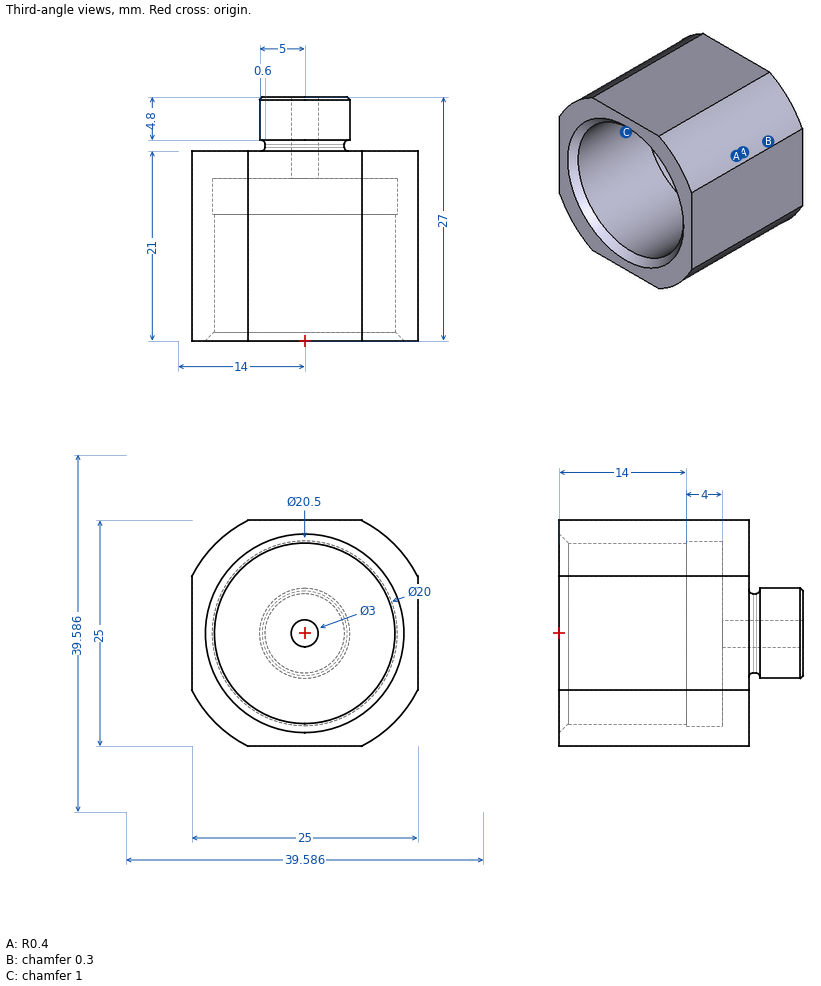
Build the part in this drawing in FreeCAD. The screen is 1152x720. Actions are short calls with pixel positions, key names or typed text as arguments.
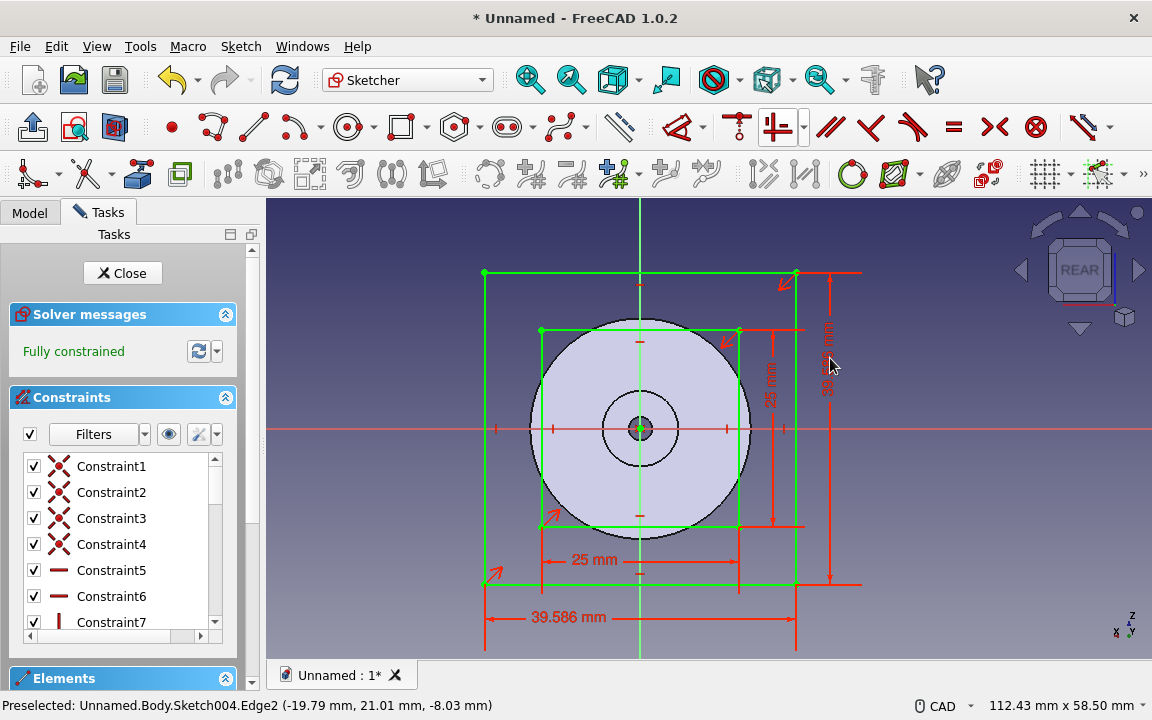
click(123, 273)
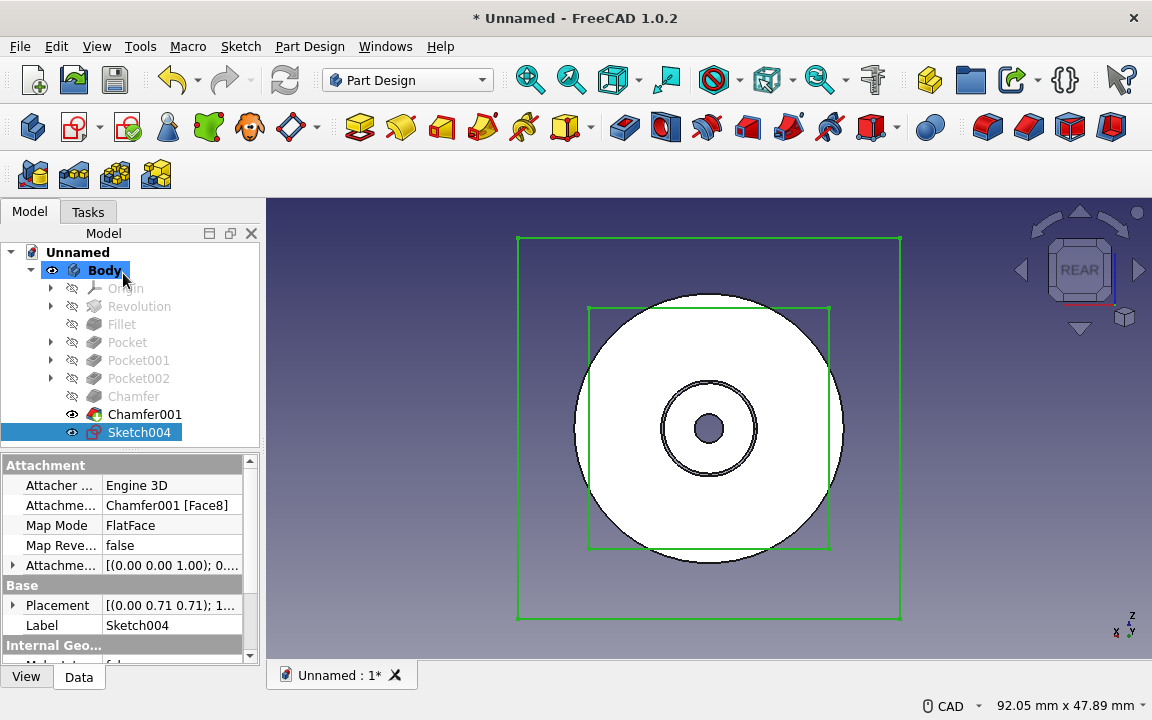
click(625, 128)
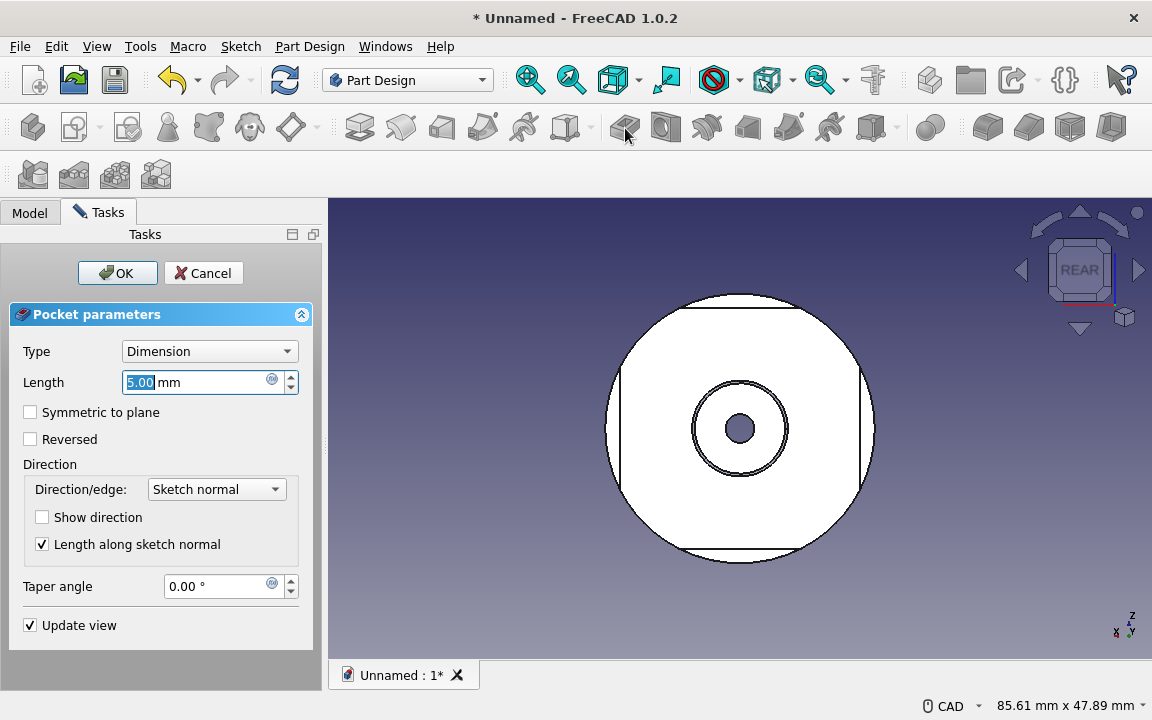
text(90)
key(Tab)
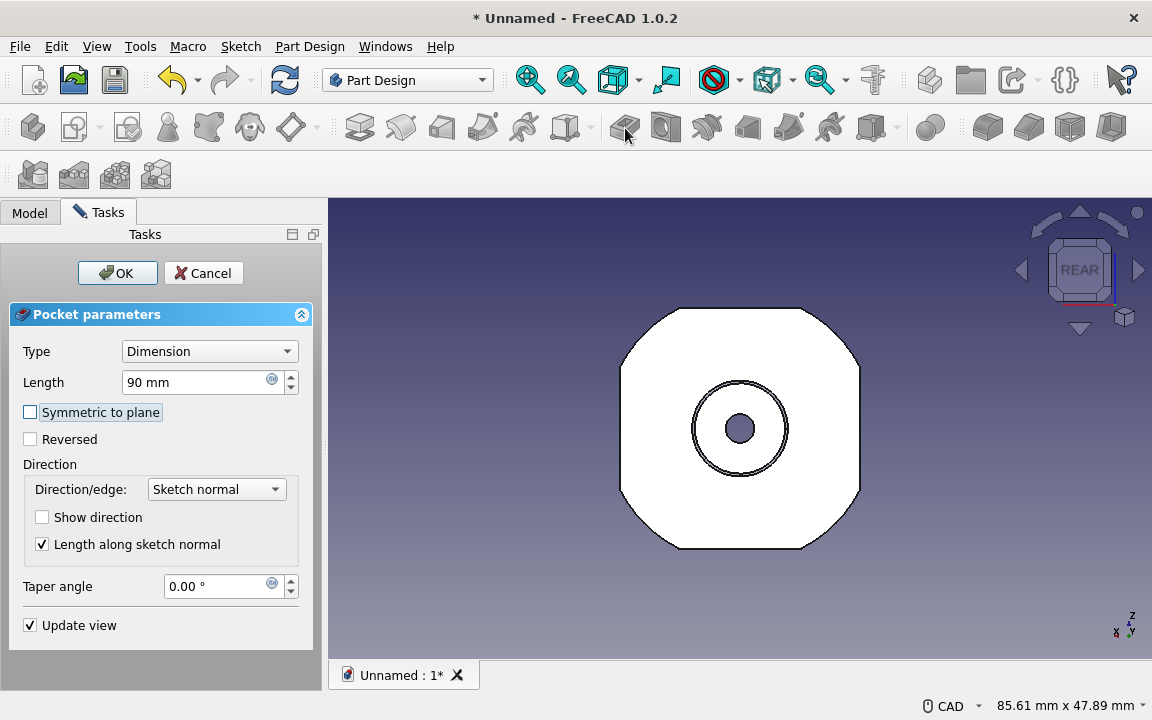
click(118, 273)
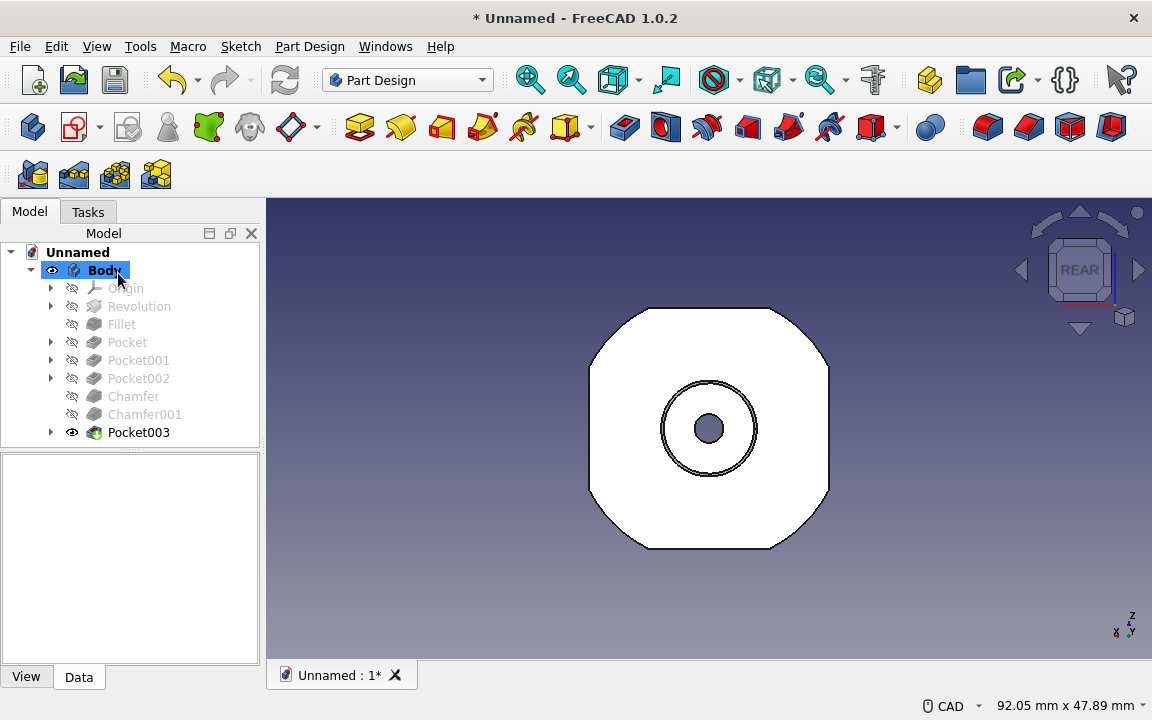
key(0)